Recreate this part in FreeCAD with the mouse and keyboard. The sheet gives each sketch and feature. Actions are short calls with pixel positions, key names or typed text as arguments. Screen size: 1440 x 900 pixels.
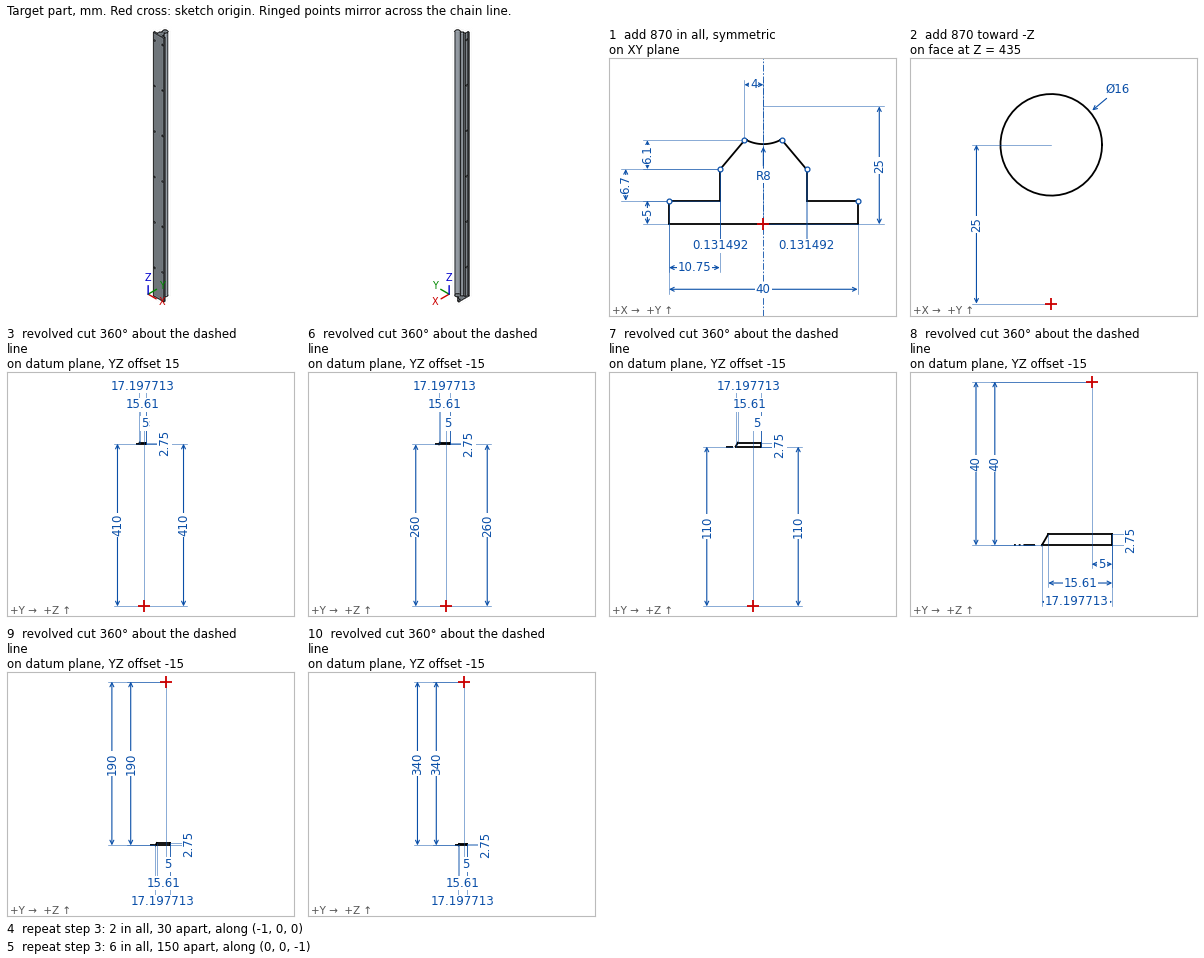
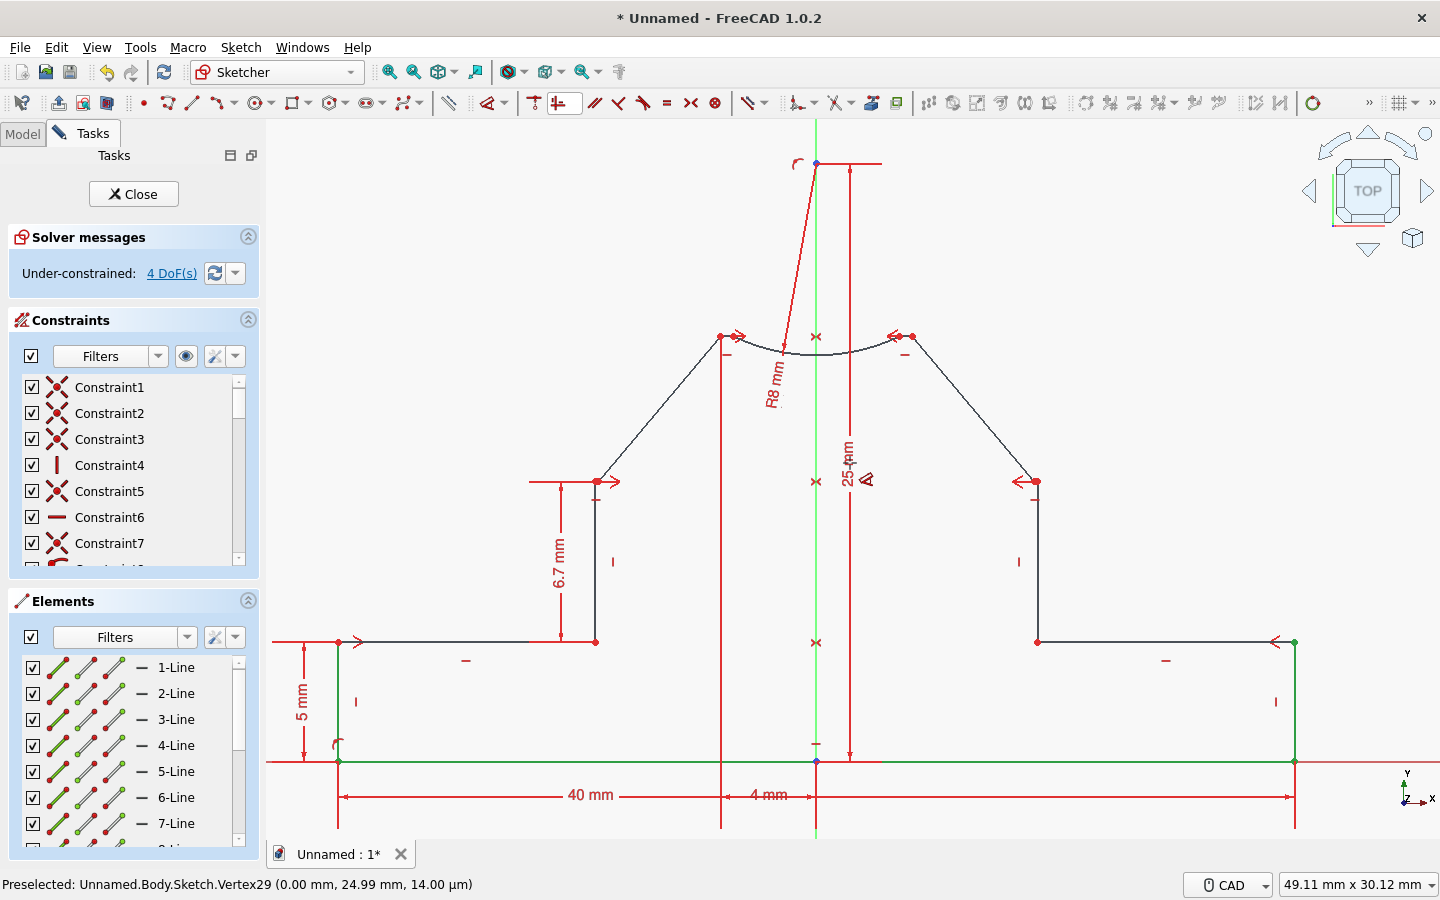
click(684, 380)
click(564, 409)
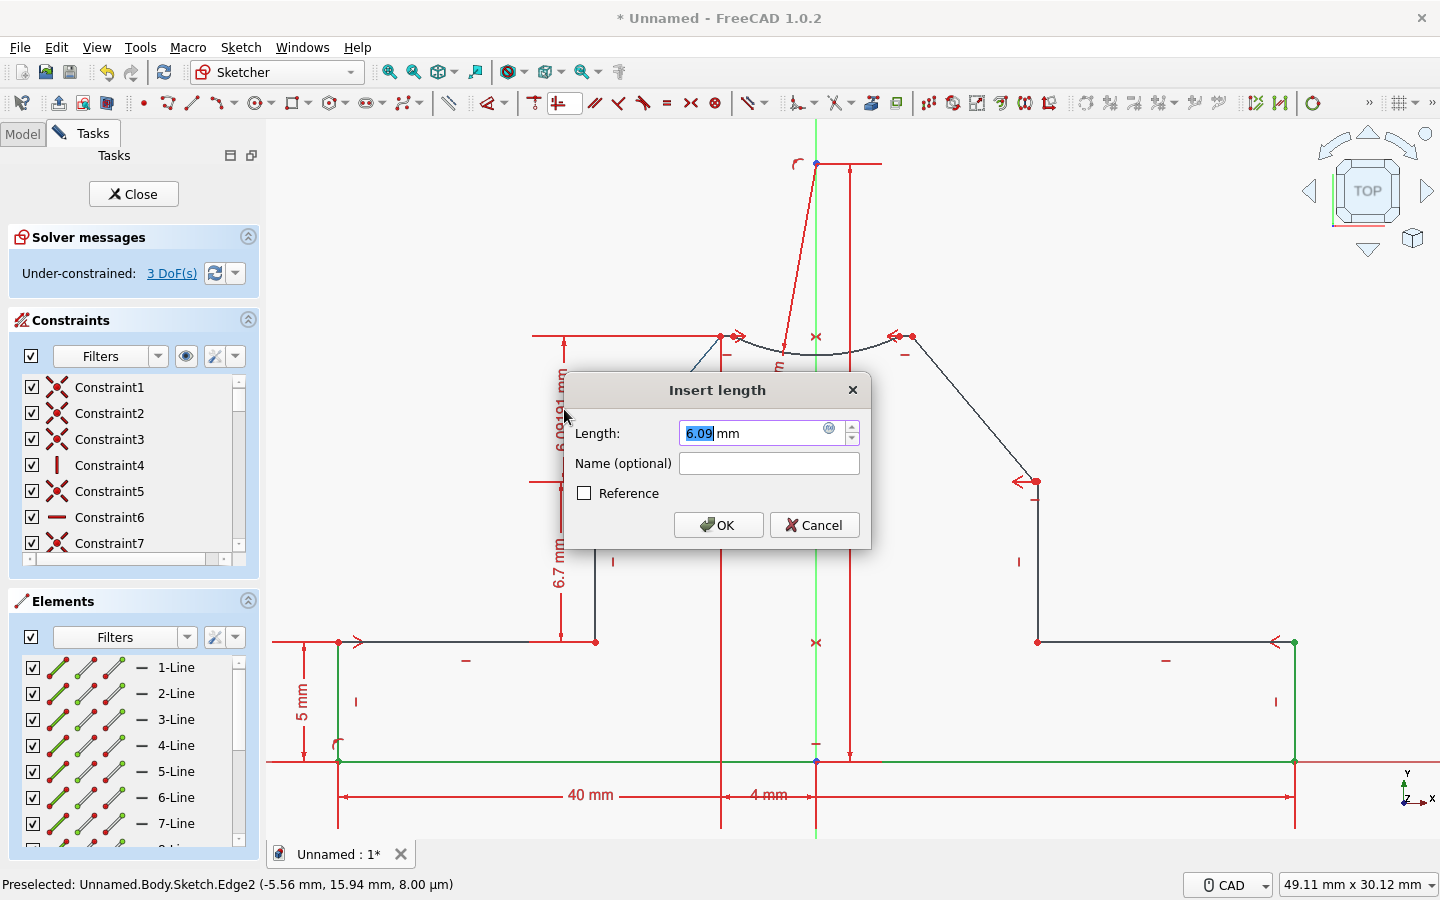
text(6.1)
key(Return)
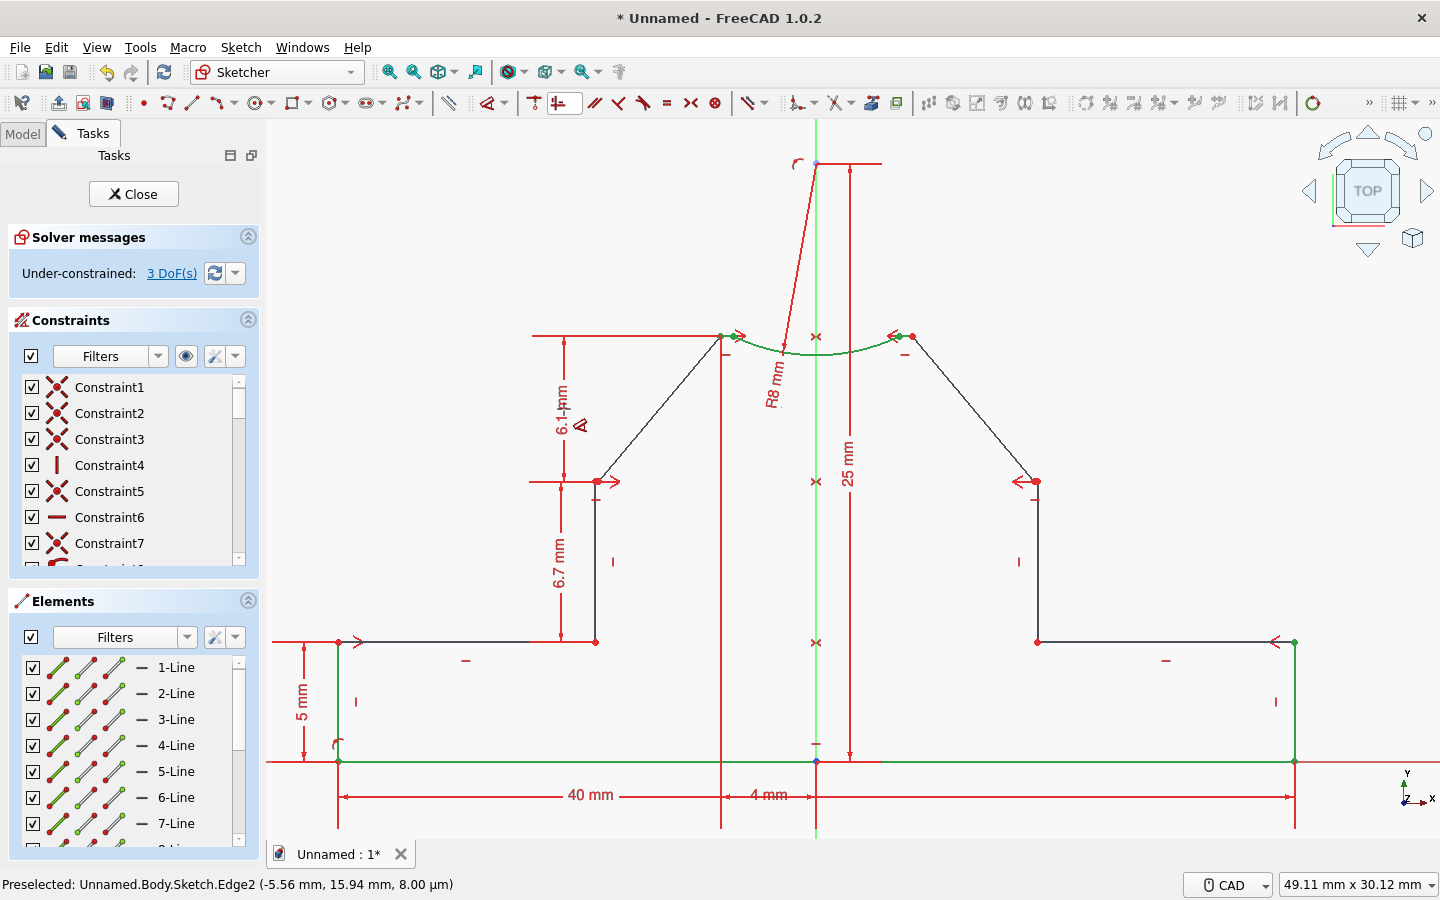
click(518, 642)
click(467, 676)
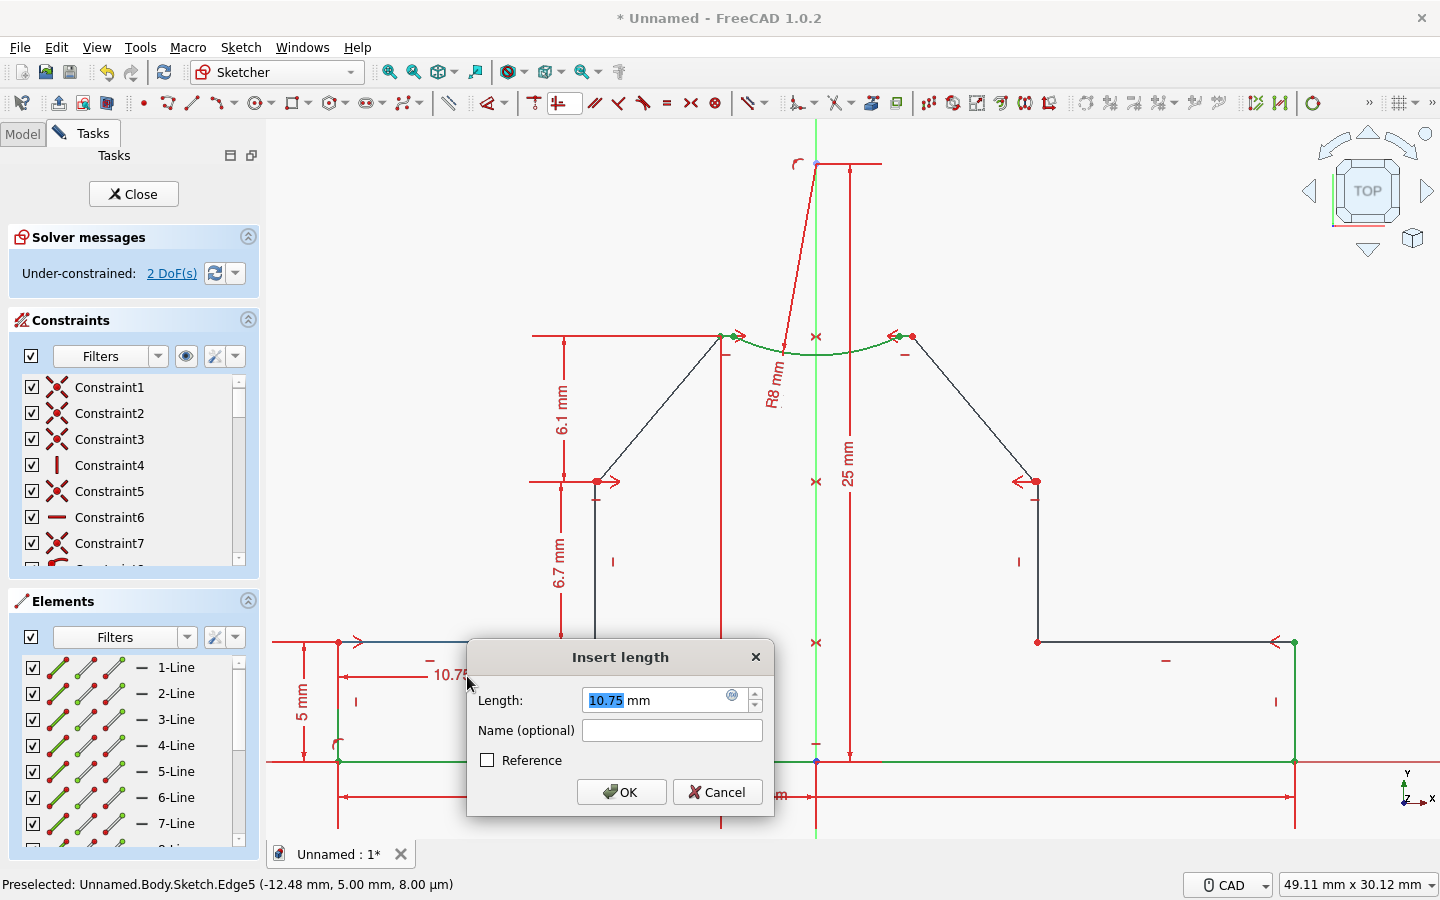
text(10.75)
key(Return)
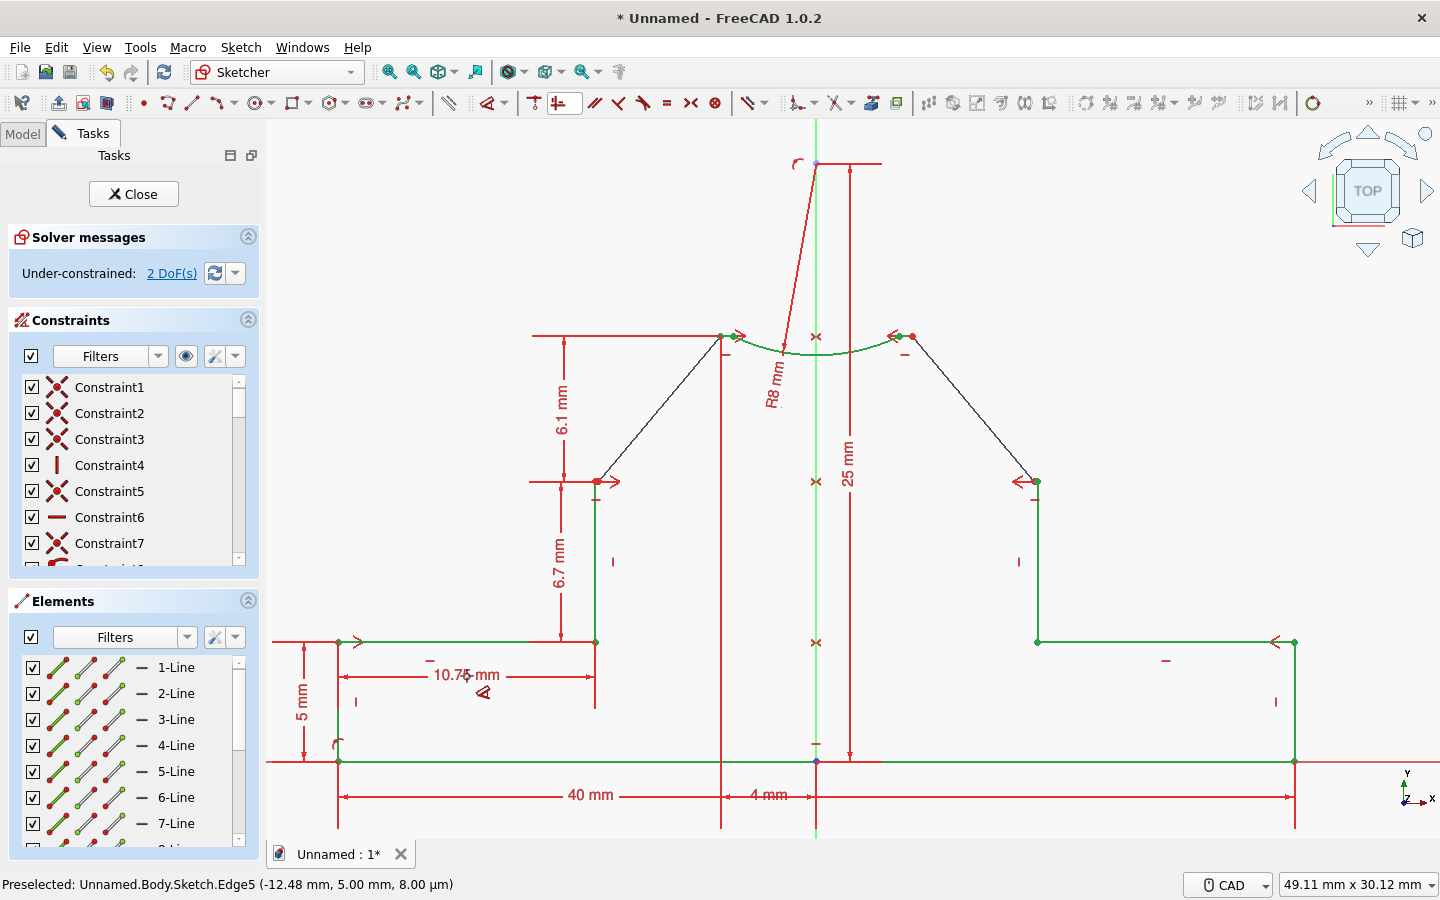
scroll(597, 482, up, 13)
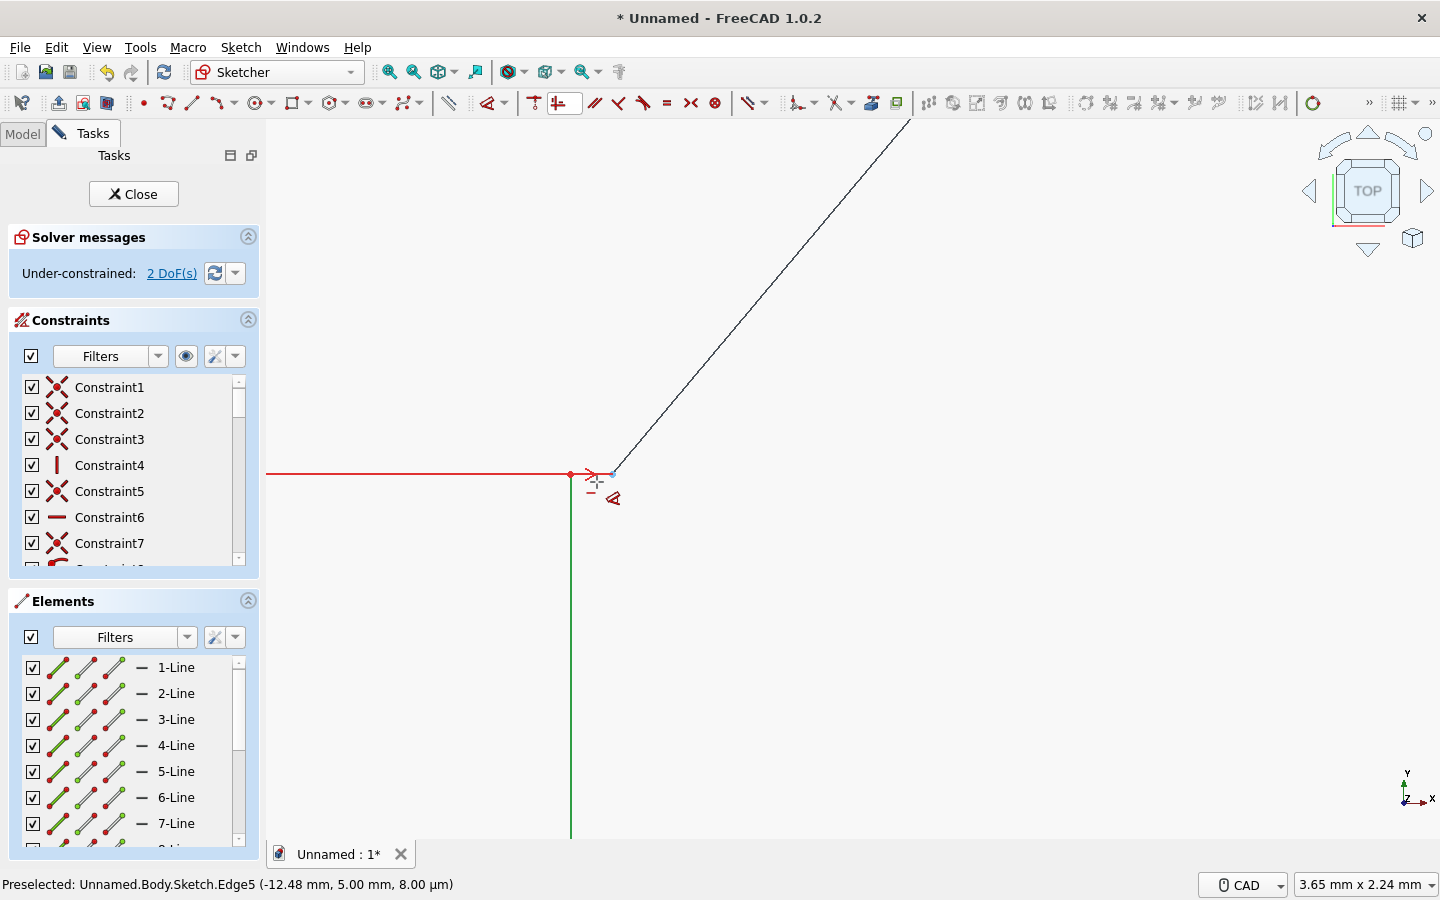
click(591, 474)
click(591, 440)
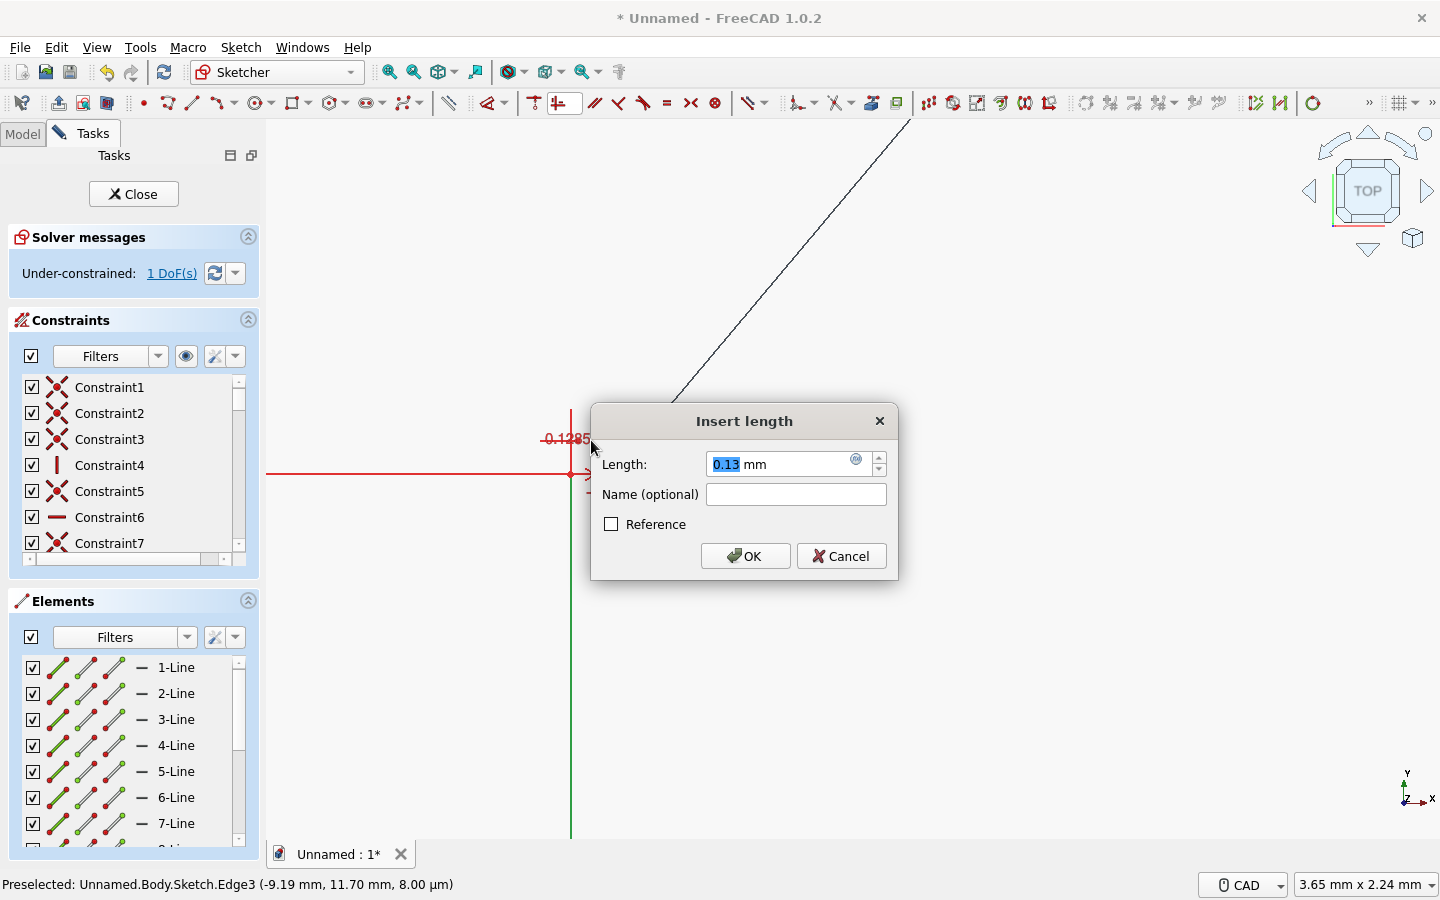
text(0.131492)
key(Return)